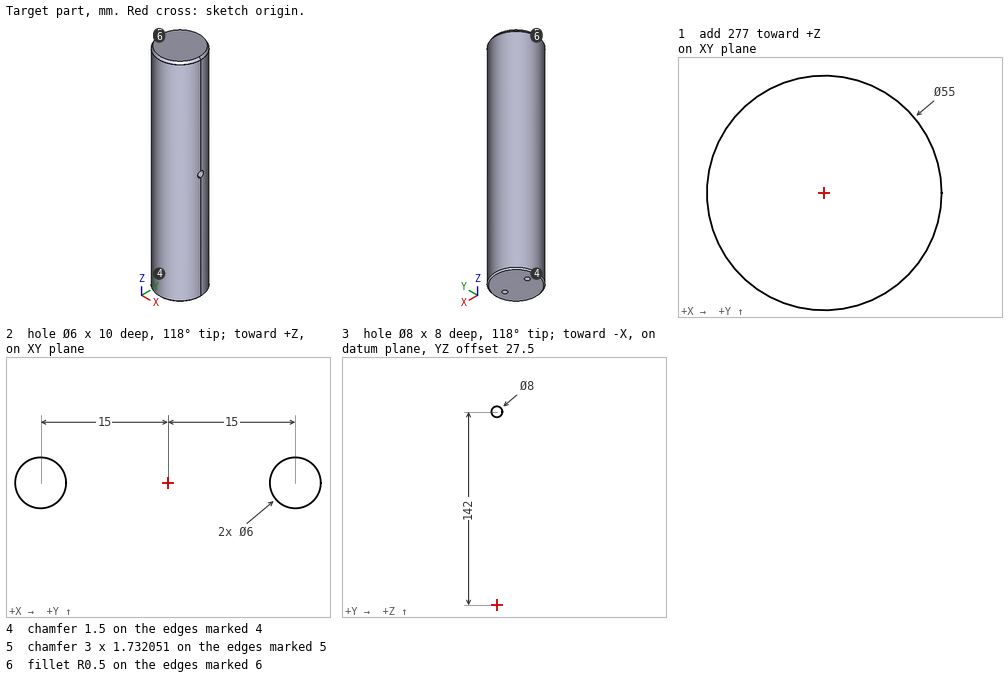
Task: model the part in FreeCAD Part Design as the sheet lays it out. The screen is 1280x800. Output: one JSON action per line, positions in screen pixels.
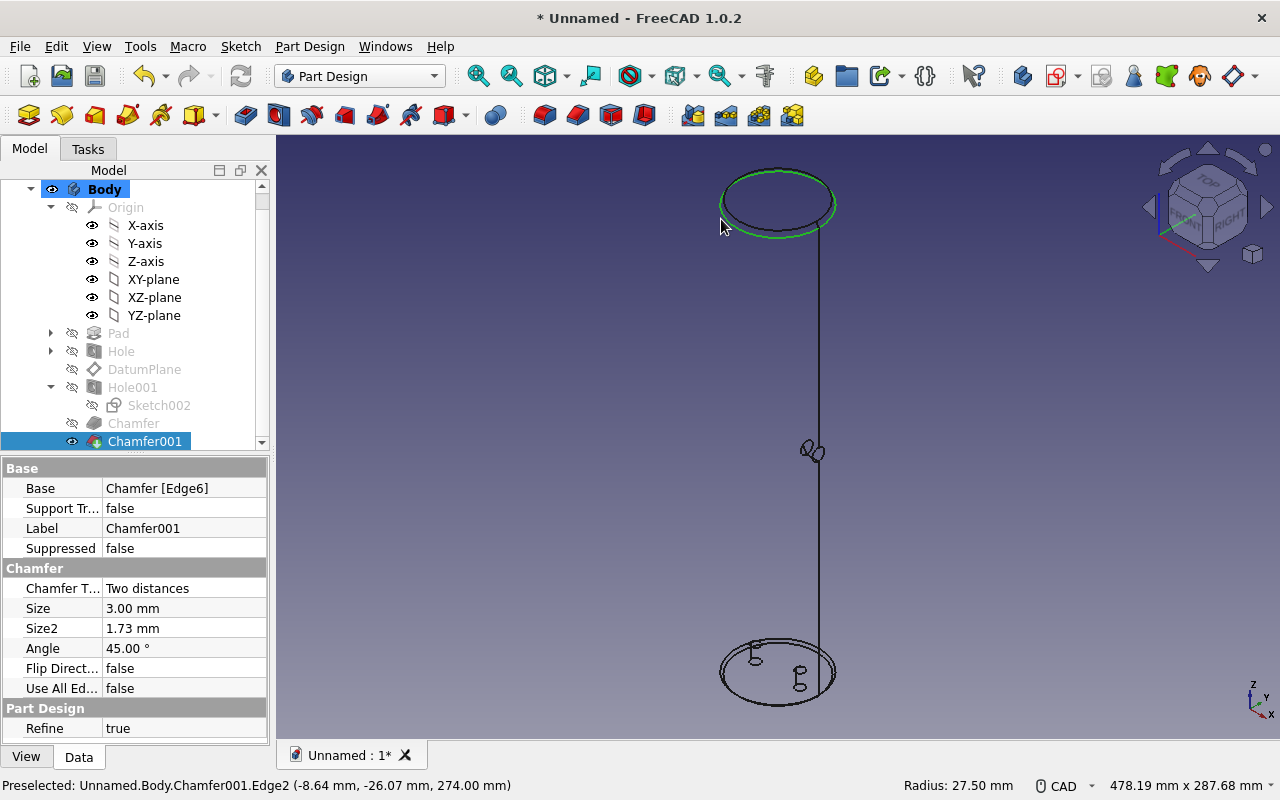
{"action": "left_click", "coordinate": [545, 116]}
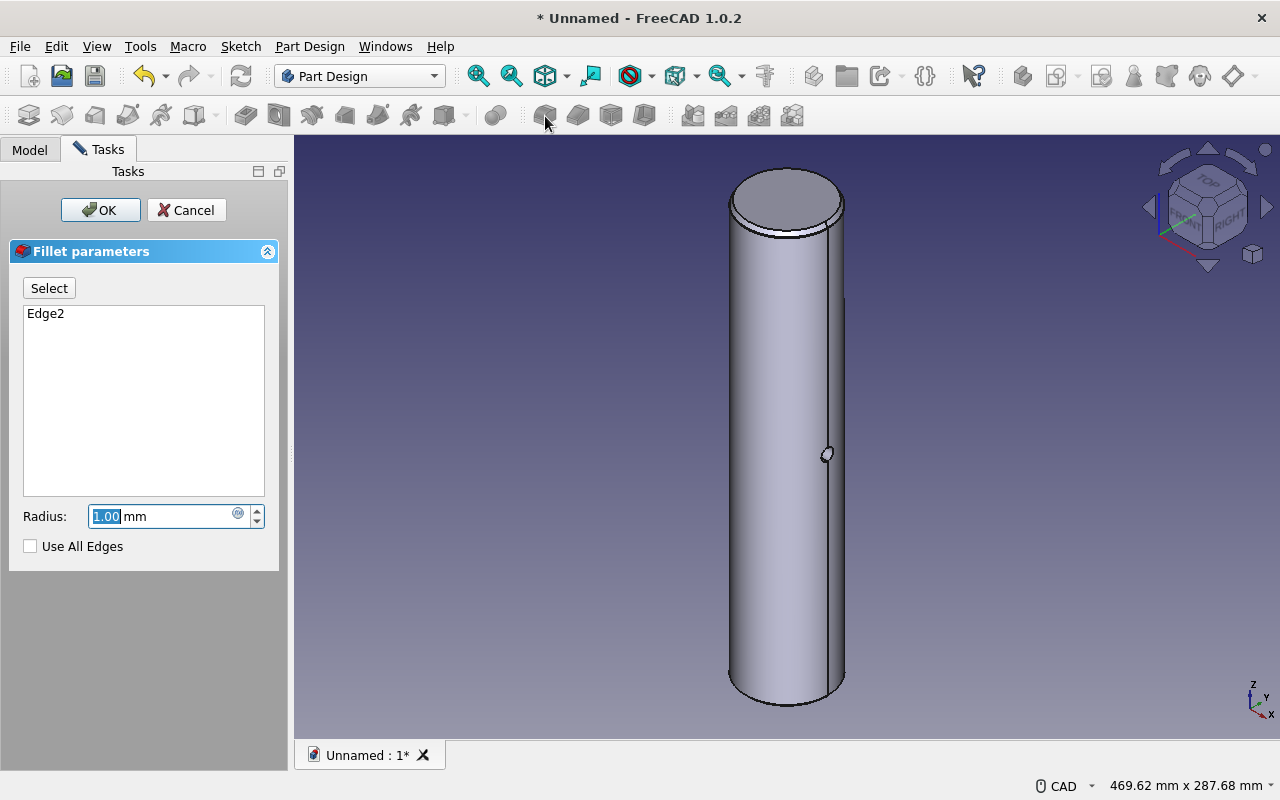
{"action": "type", "text": "0.5"}
{"action": "key", "text": "Tab"}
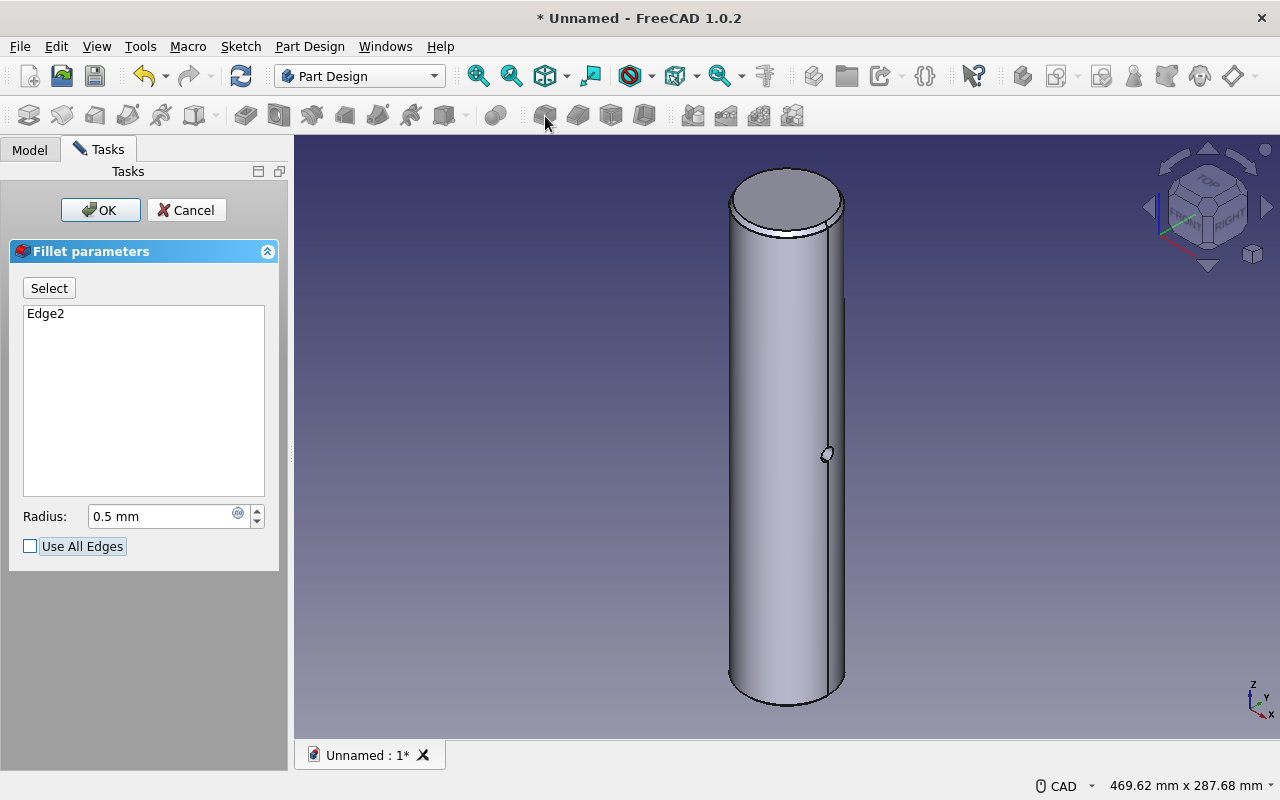
{"action": "left_click", "coordinate": [101, 210]}